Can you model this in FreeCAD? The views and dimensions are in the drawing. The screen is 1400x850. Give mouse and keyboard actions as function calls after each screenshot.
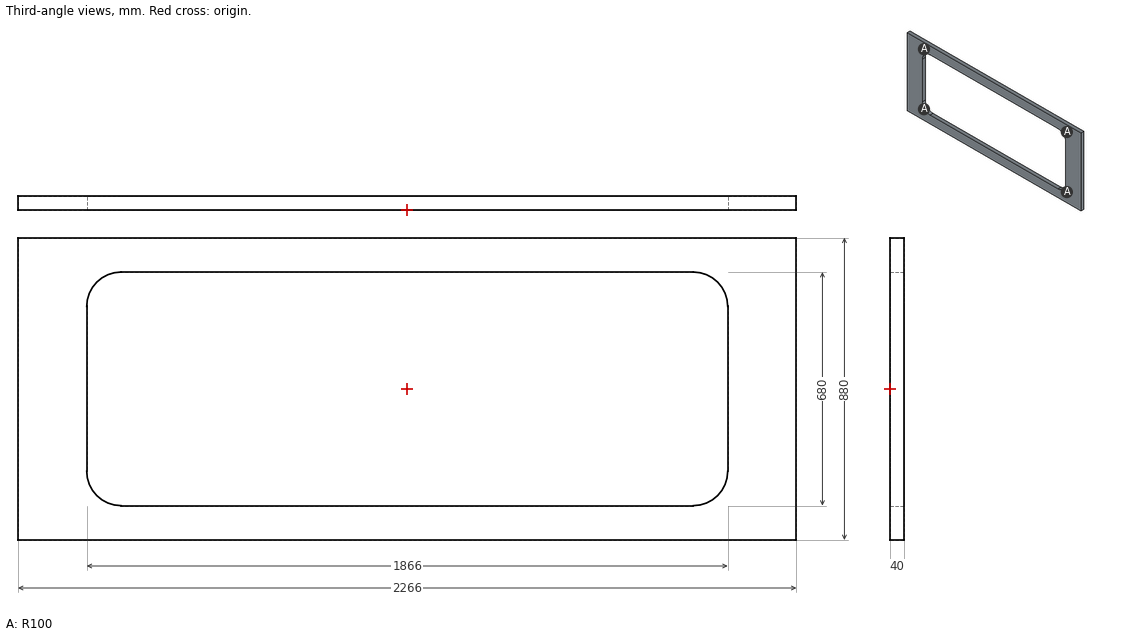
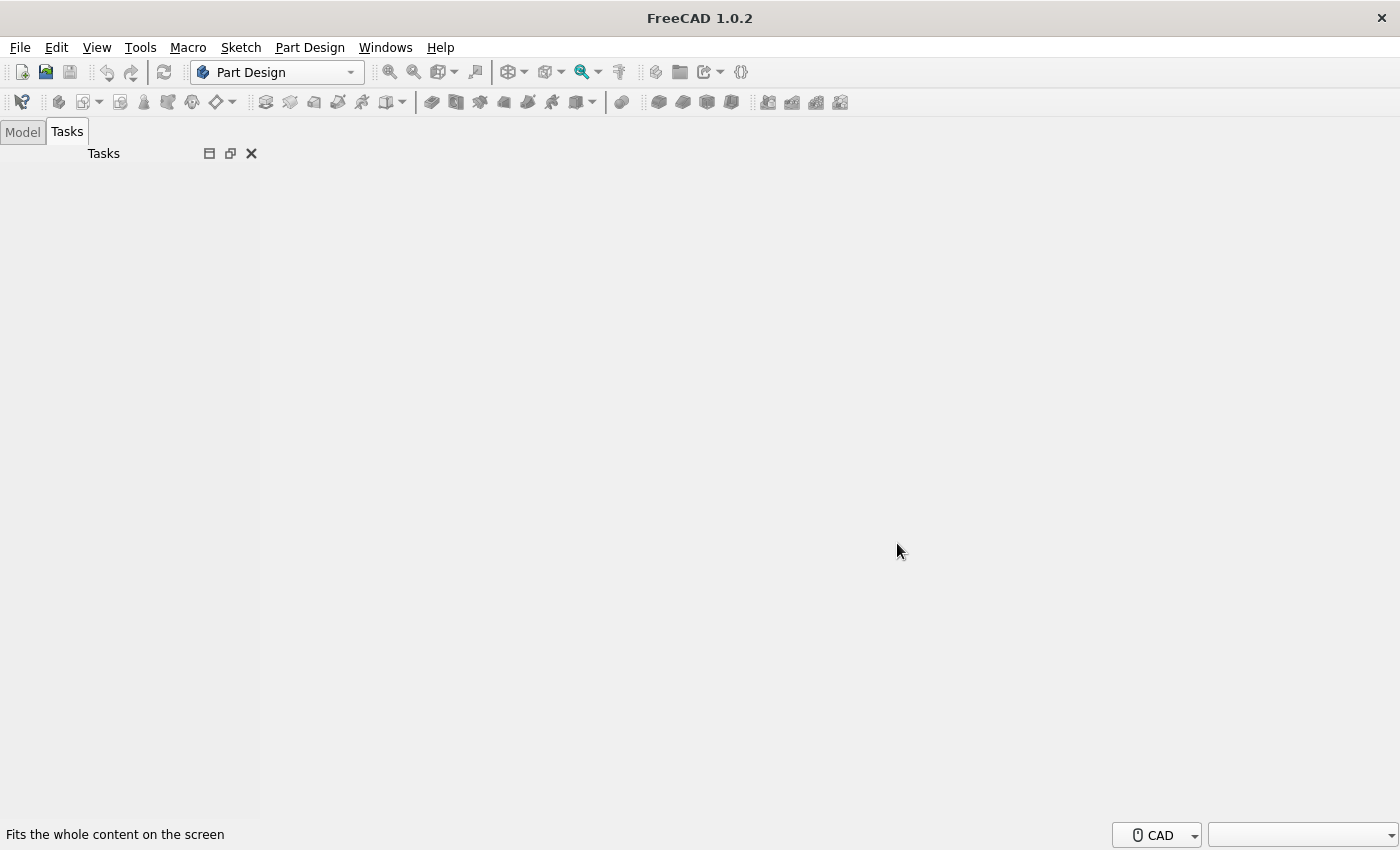
key(ctrl+n)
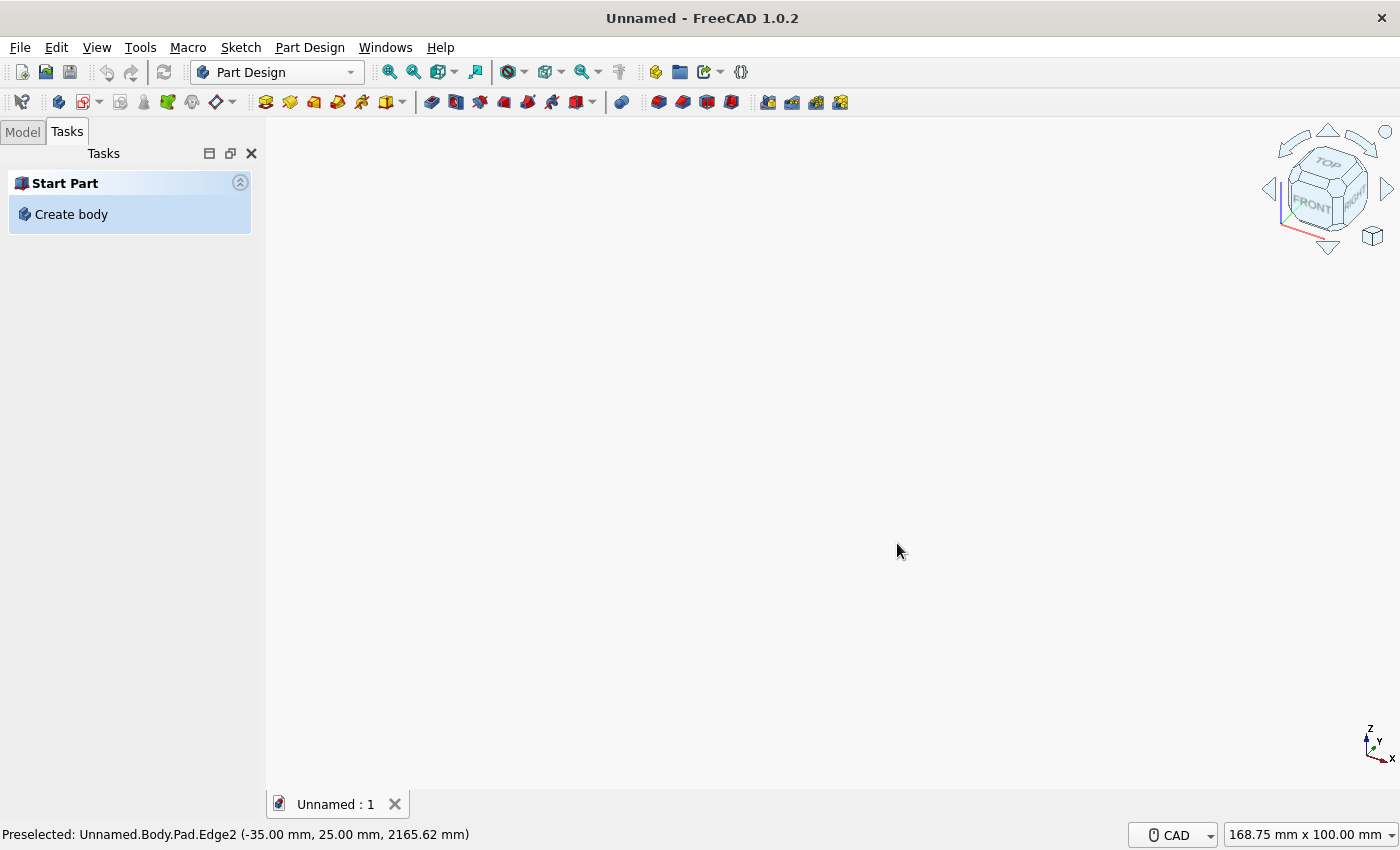
click(84, 102)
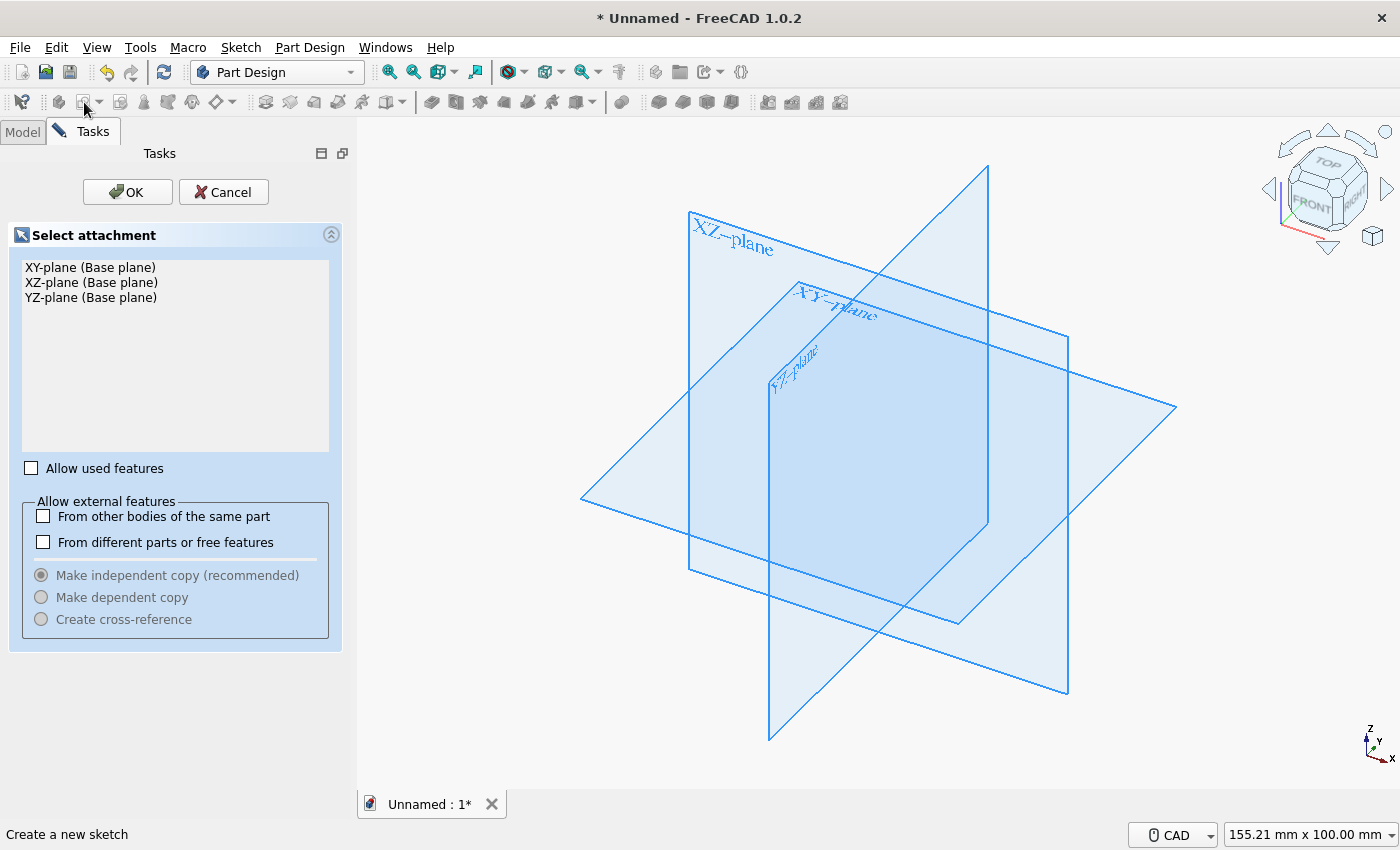
click(82, 282)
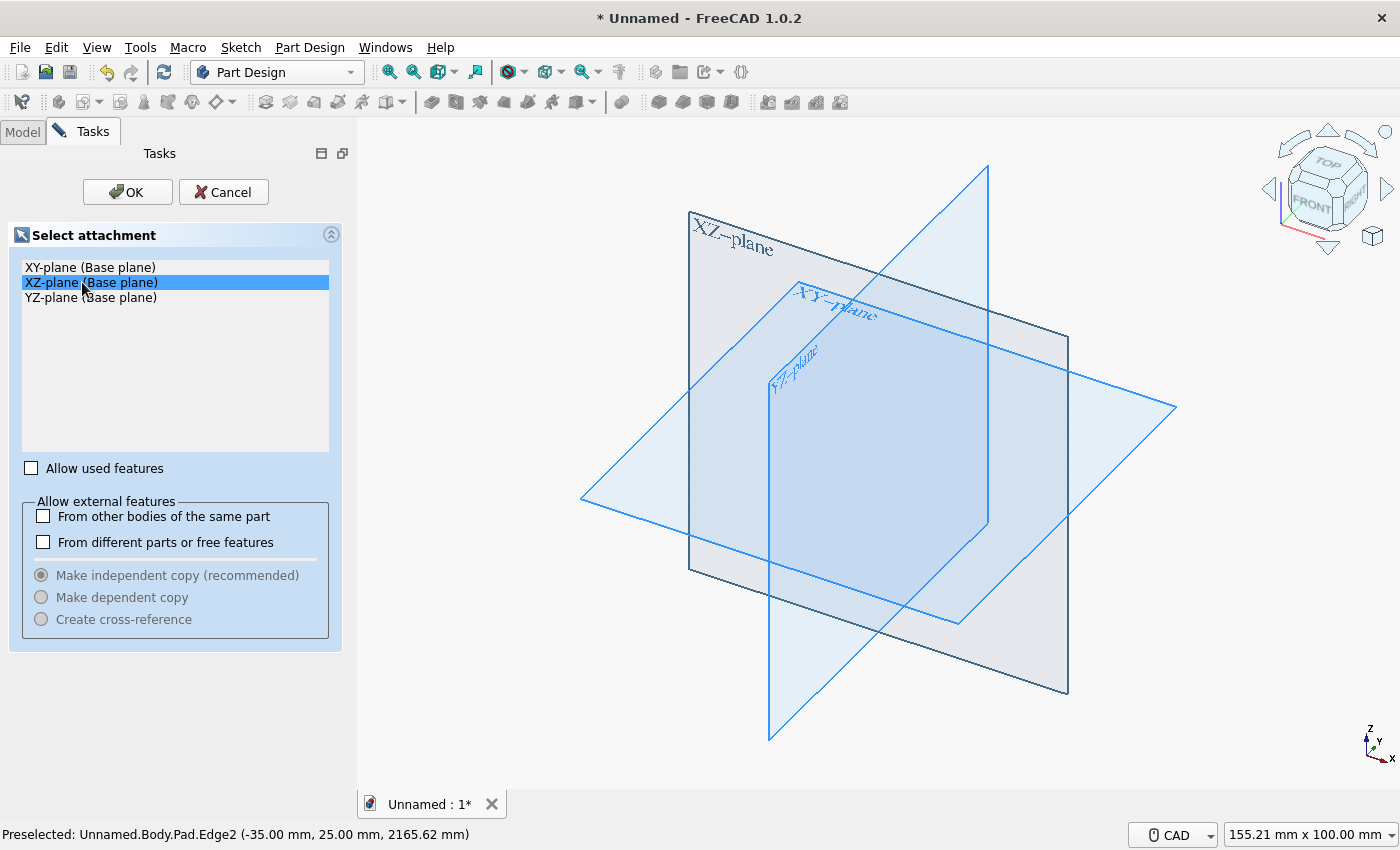
click(128, 192)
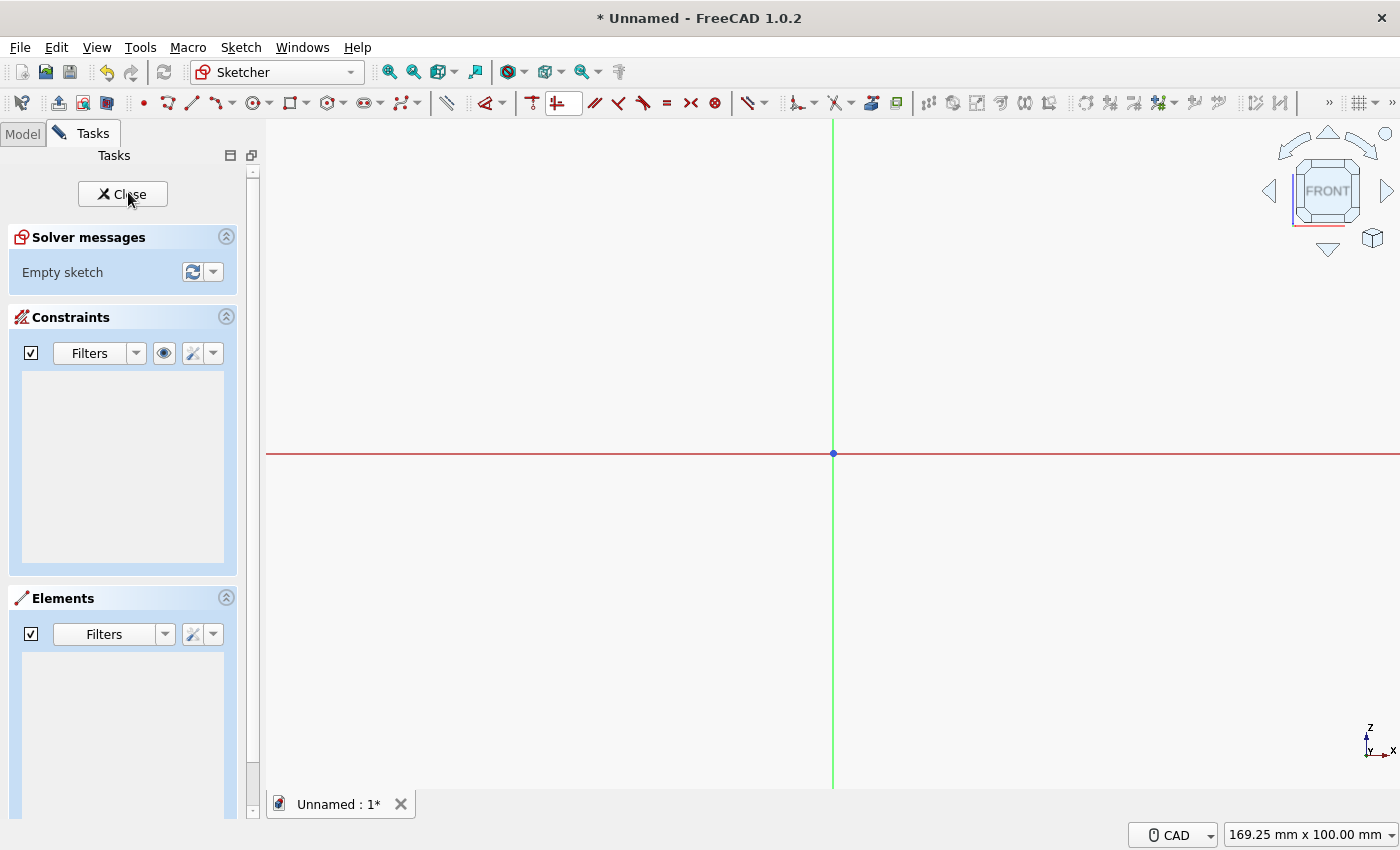
scroll(761, 454, down, 15)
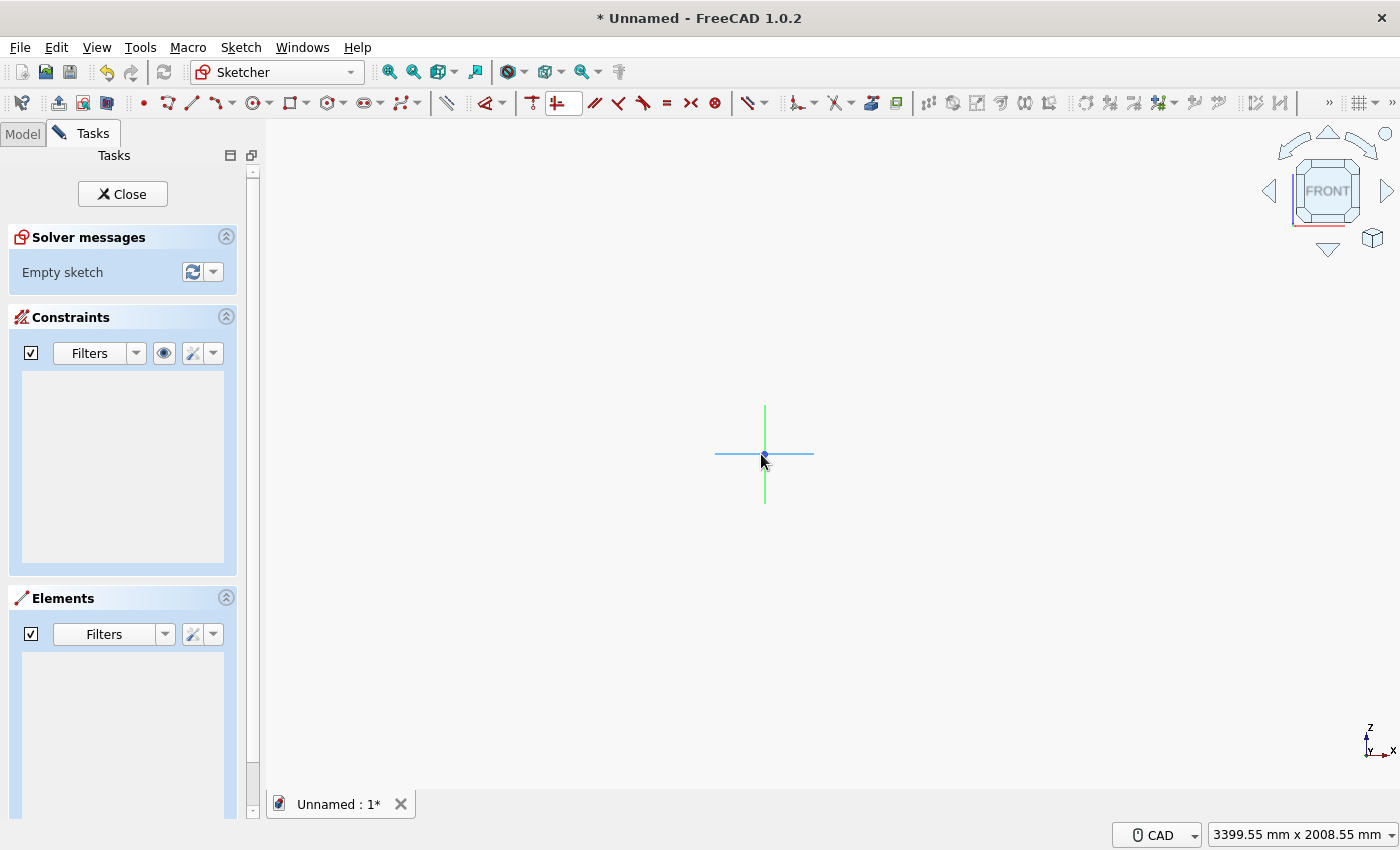
key(g)
key(v)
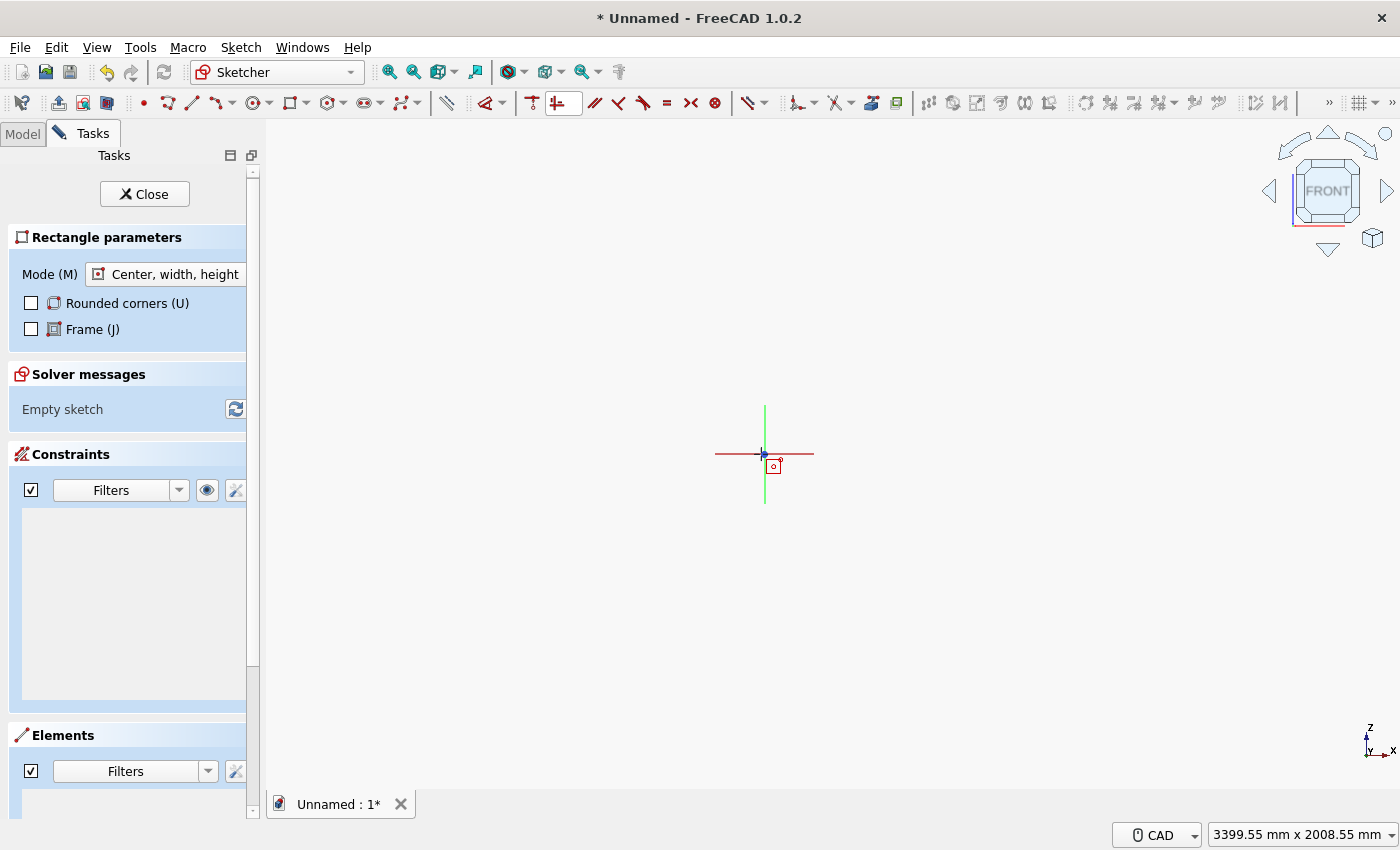
click(765, 454)
click(1143, 308)
key(Escape)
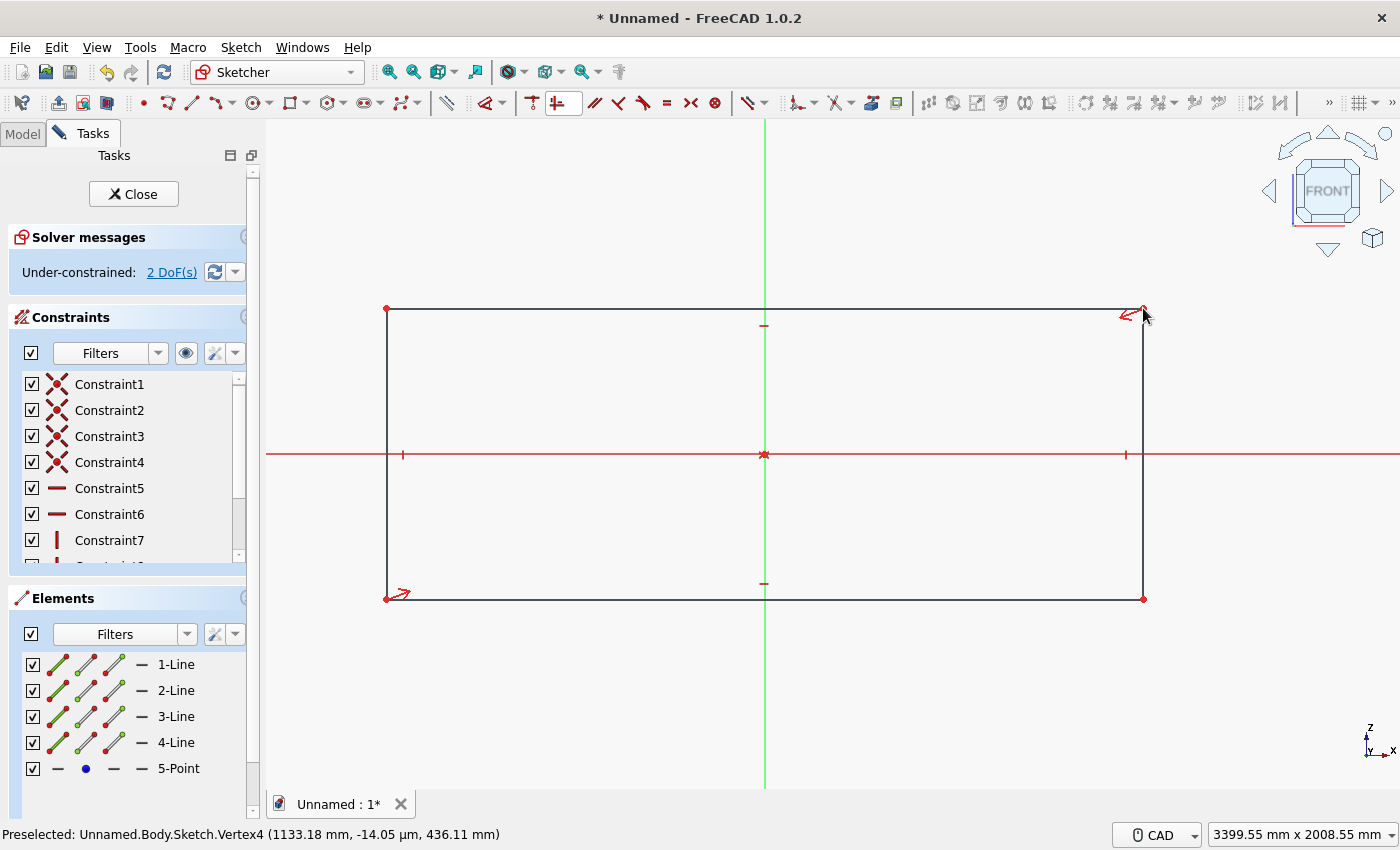
key(d)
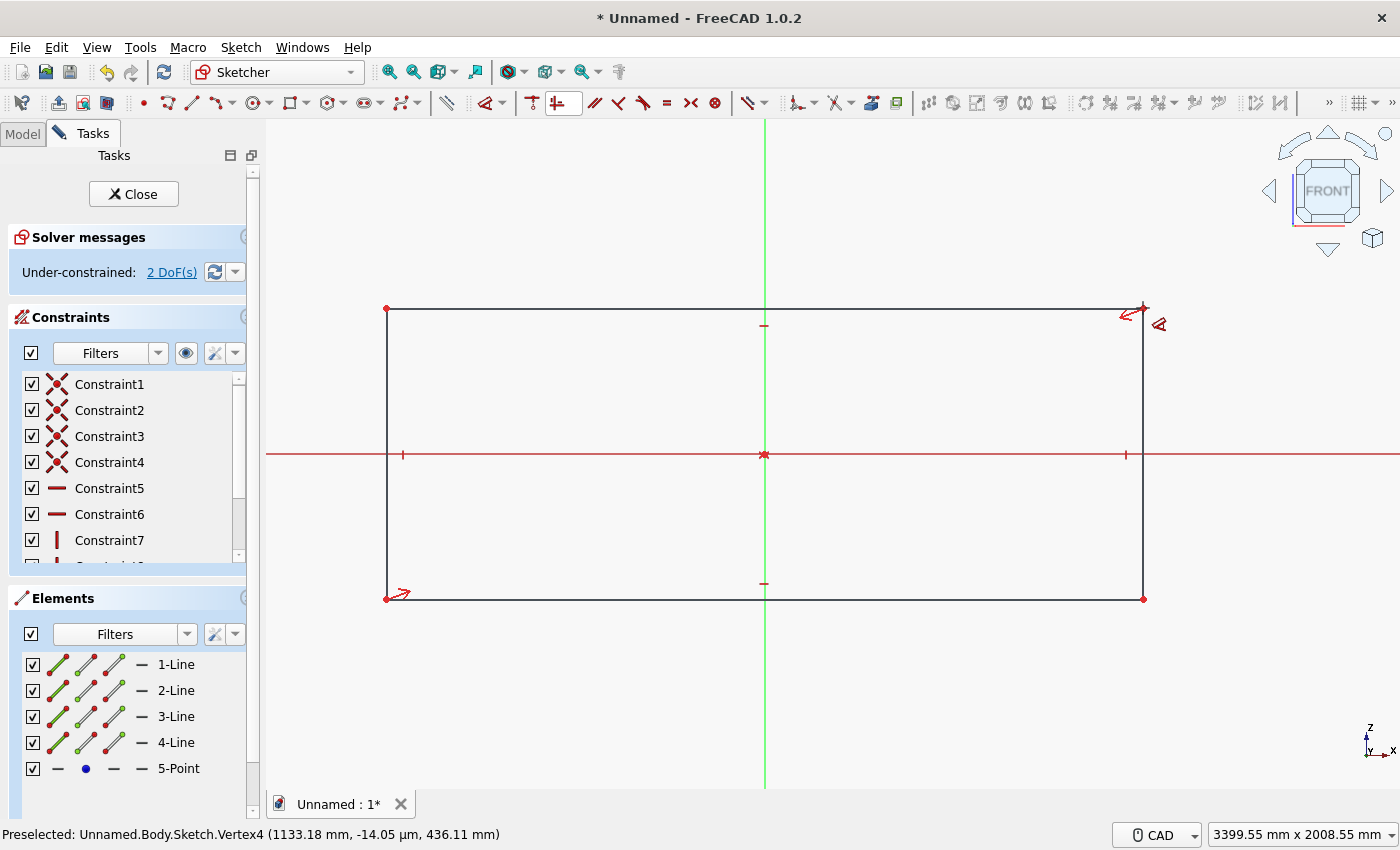
click(1143, 513)
click(1177, 388)